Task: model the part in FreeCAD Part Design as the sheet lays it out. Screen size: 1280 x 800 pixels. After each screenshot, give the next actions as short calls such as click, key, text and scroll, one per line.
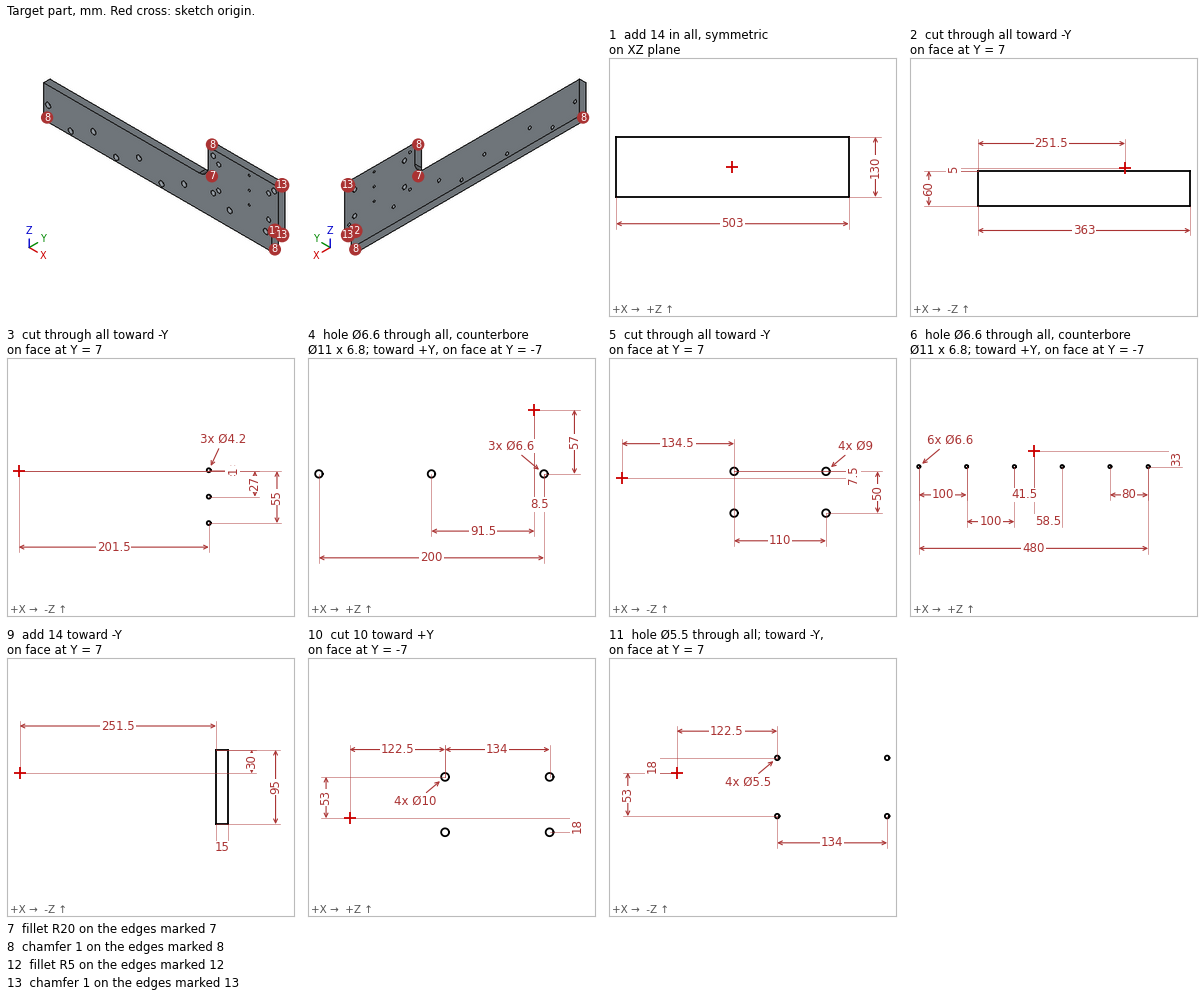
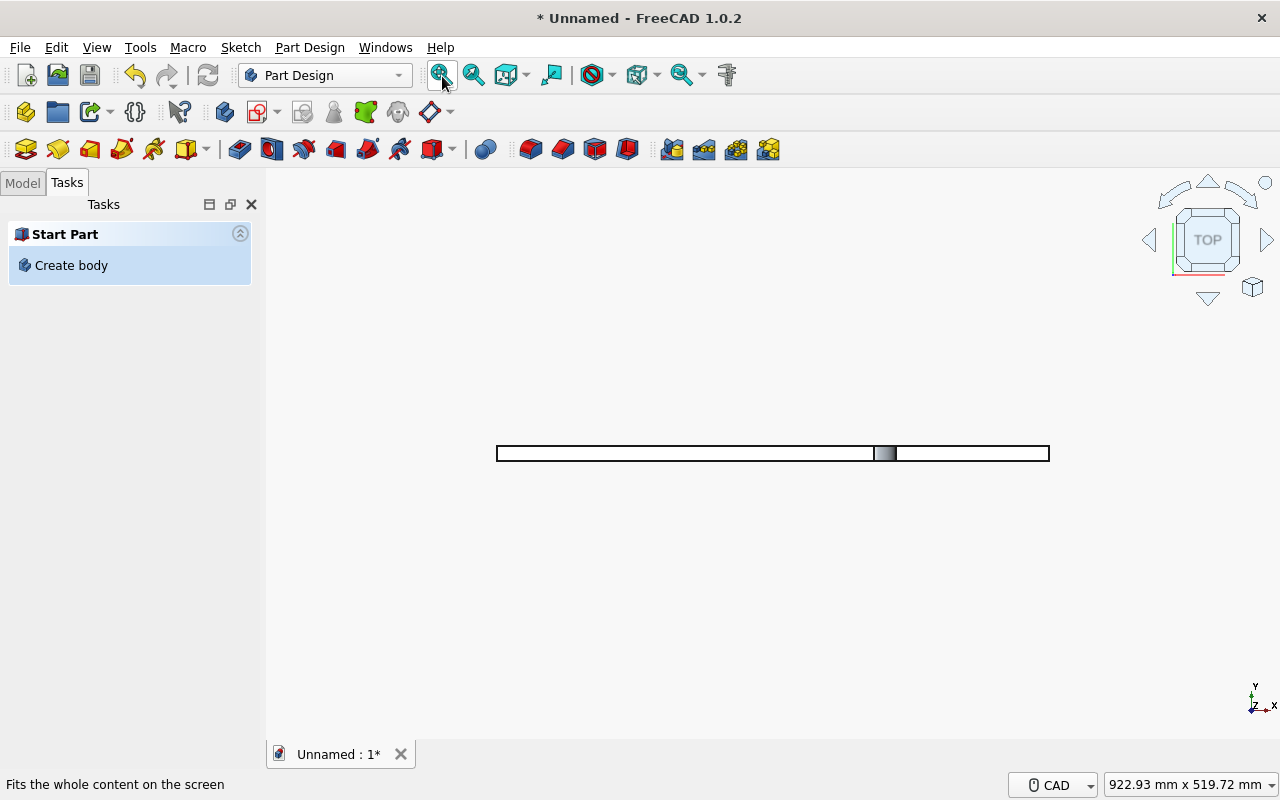
click(896, 452)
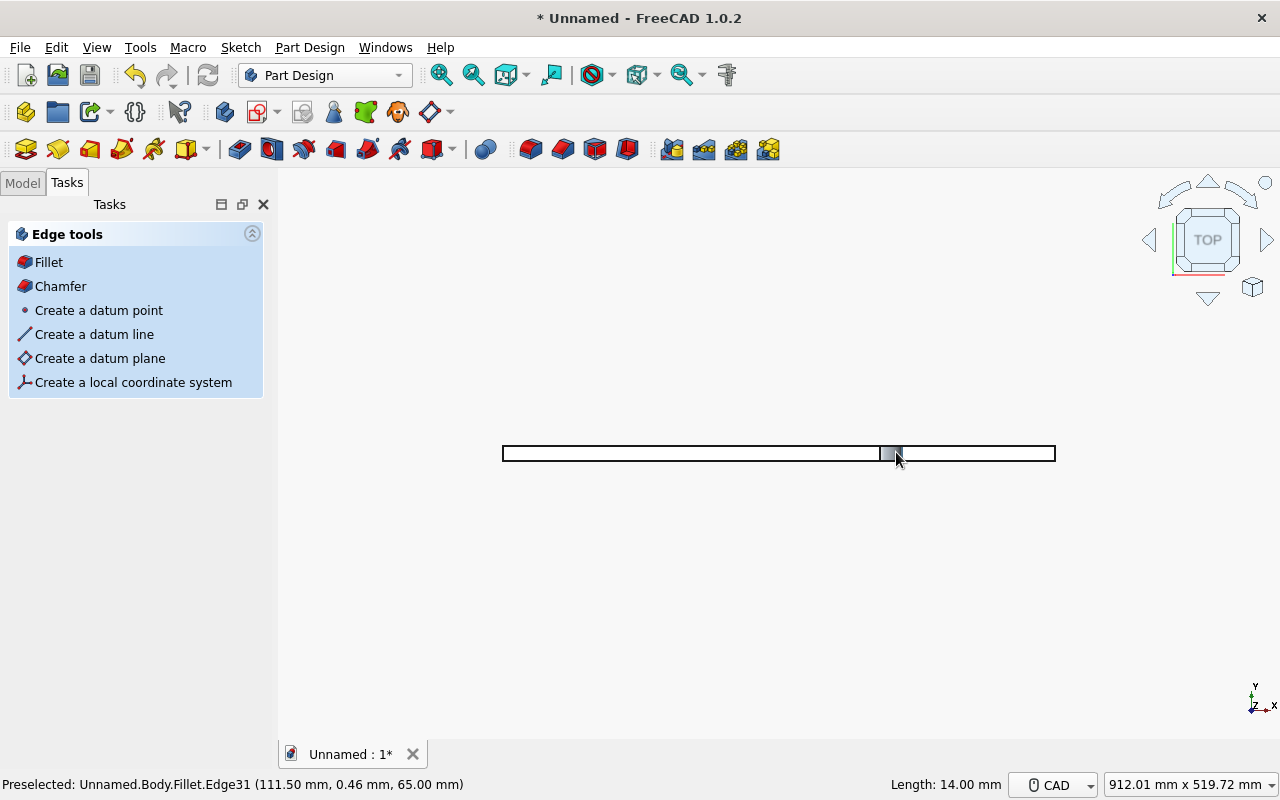
scroll(503, 452, up, 5)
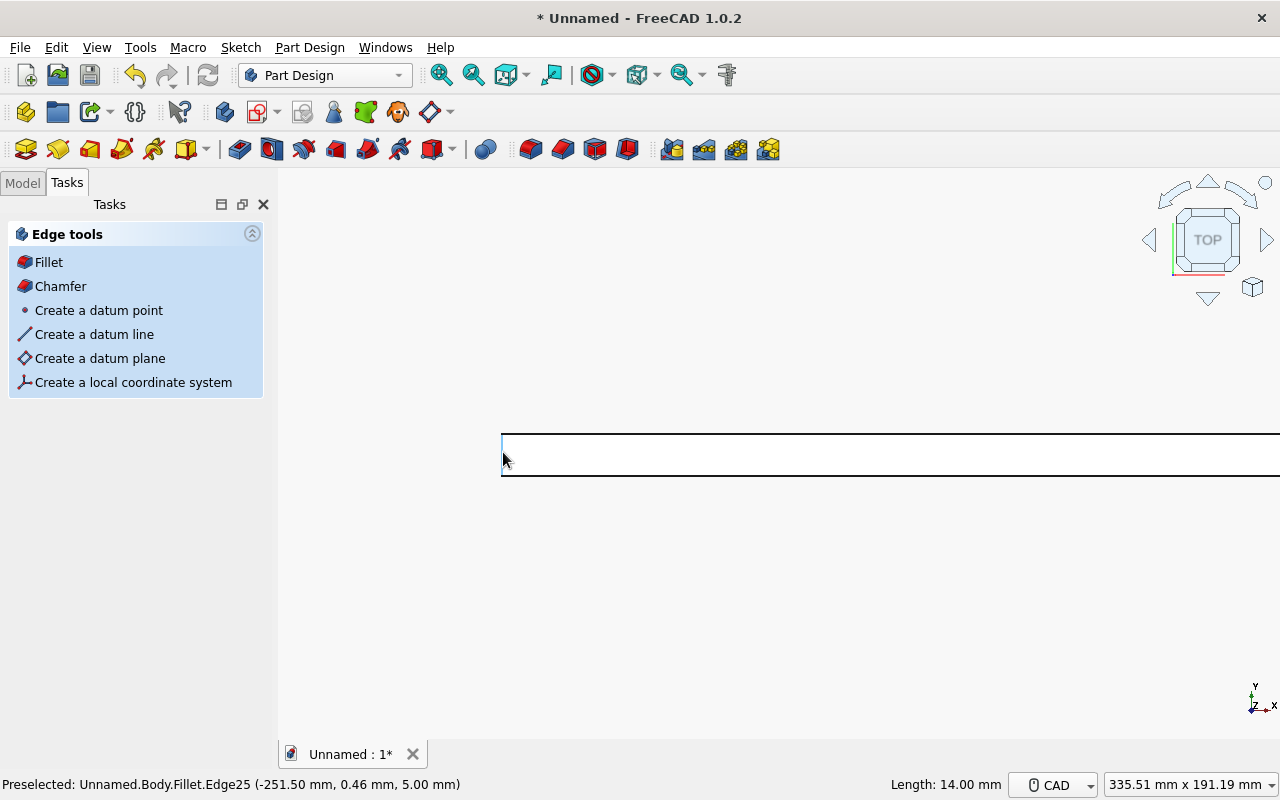
key(v)
key(f)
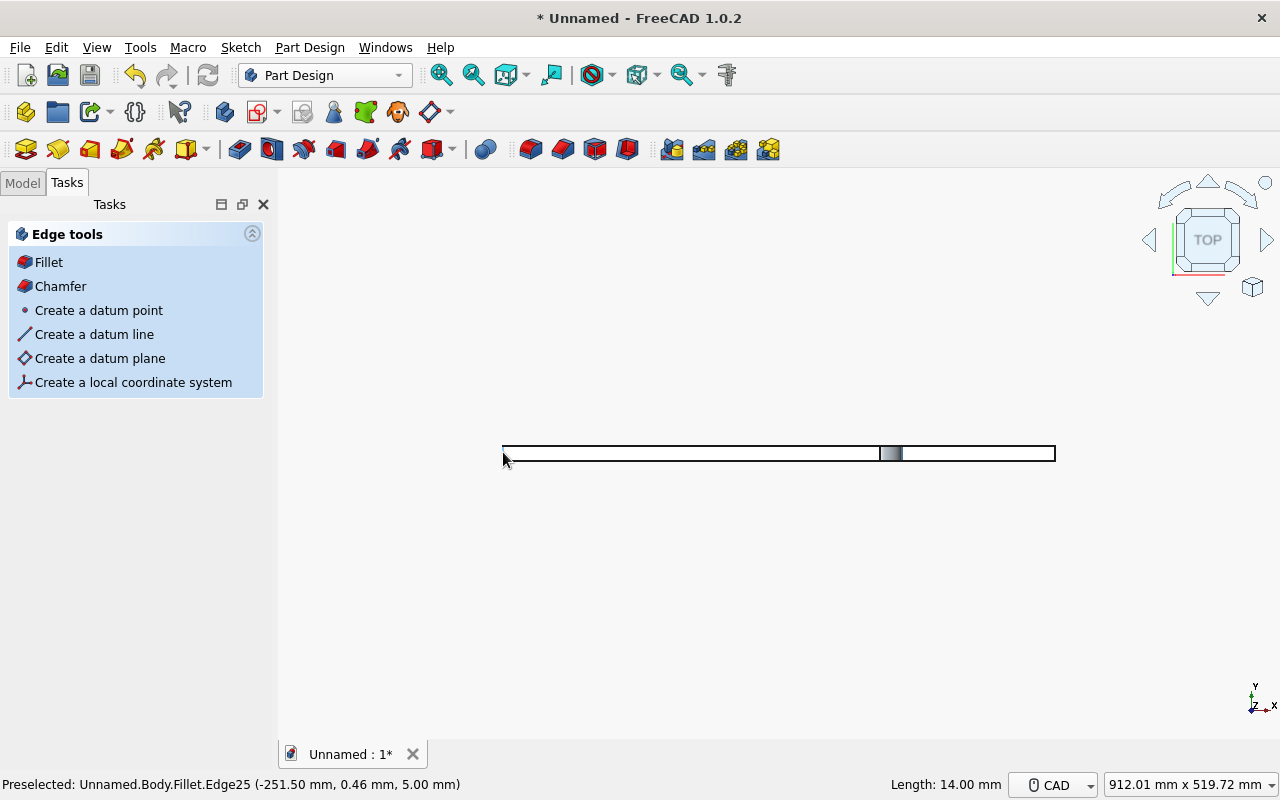
key(0)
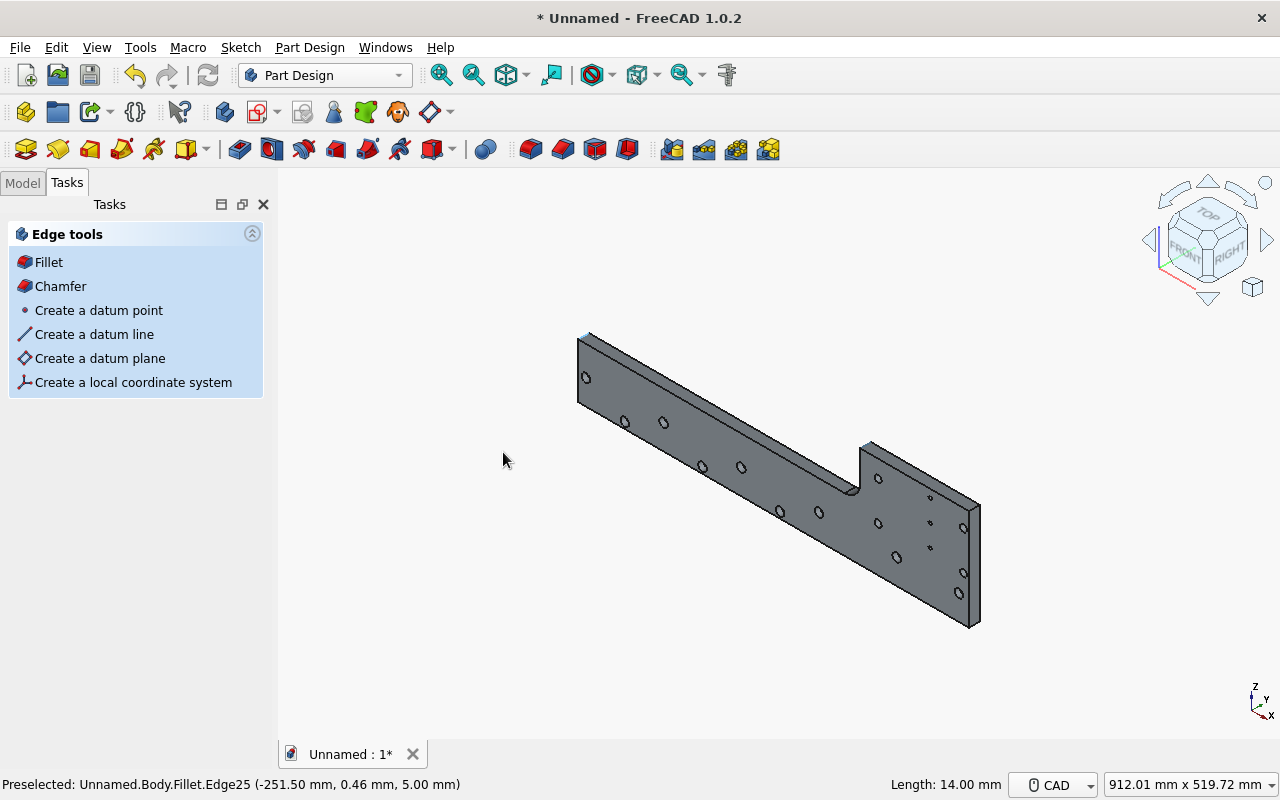
scroll(584, 398, up, 5)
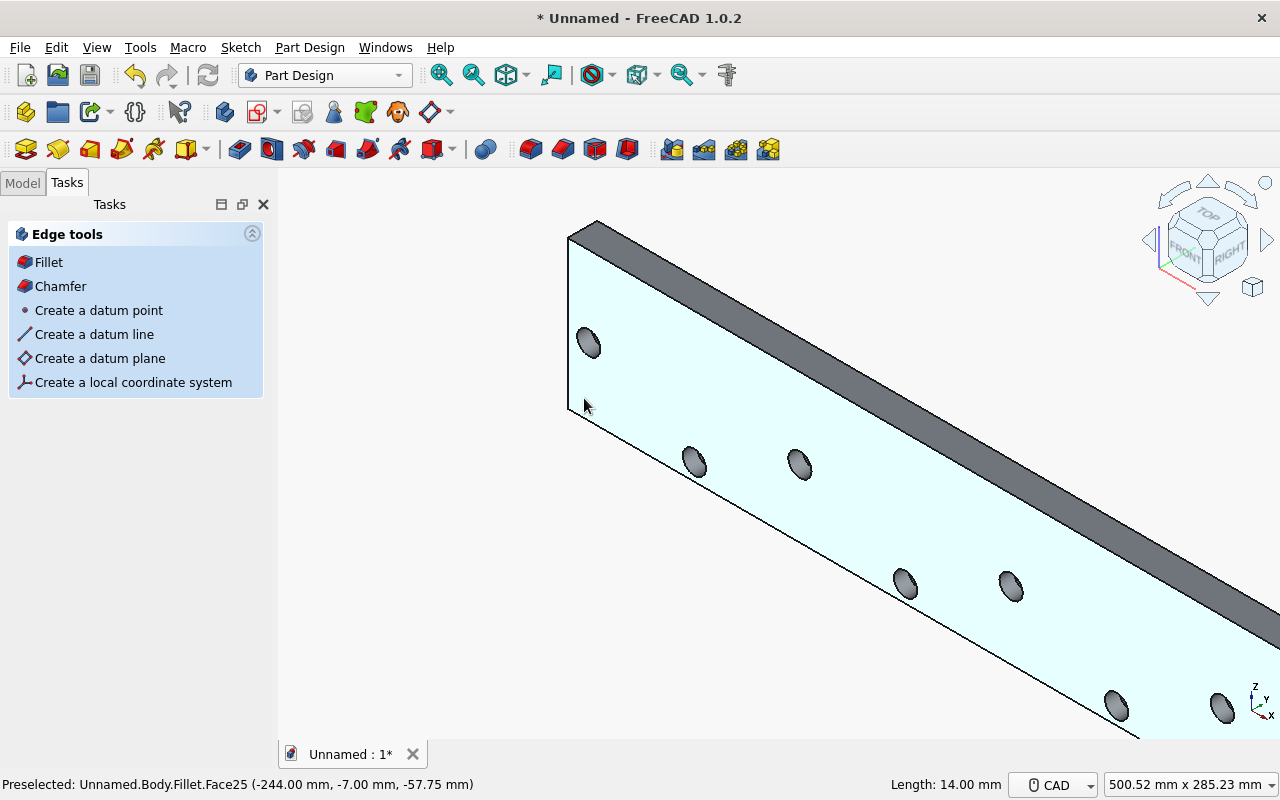
key(v)
key(f)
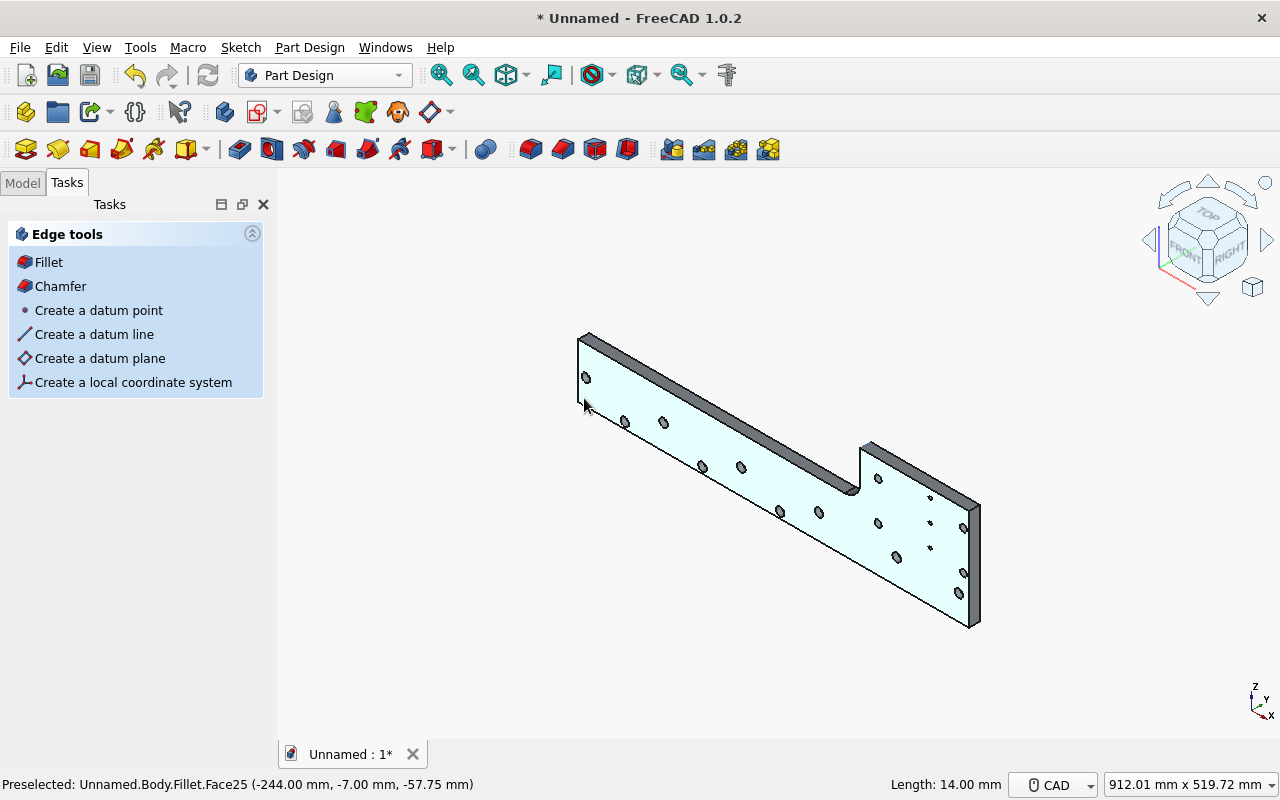
key(1)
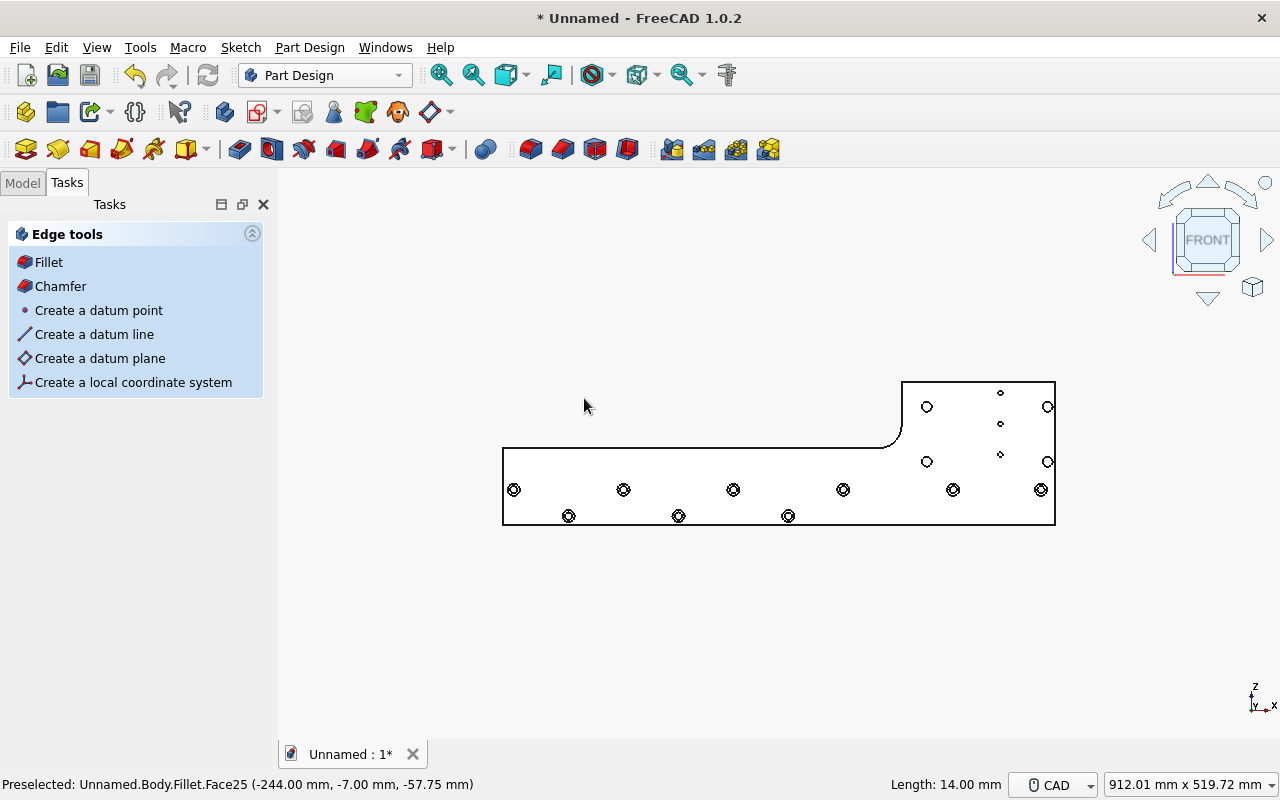
scroll(503, 524, up, 5)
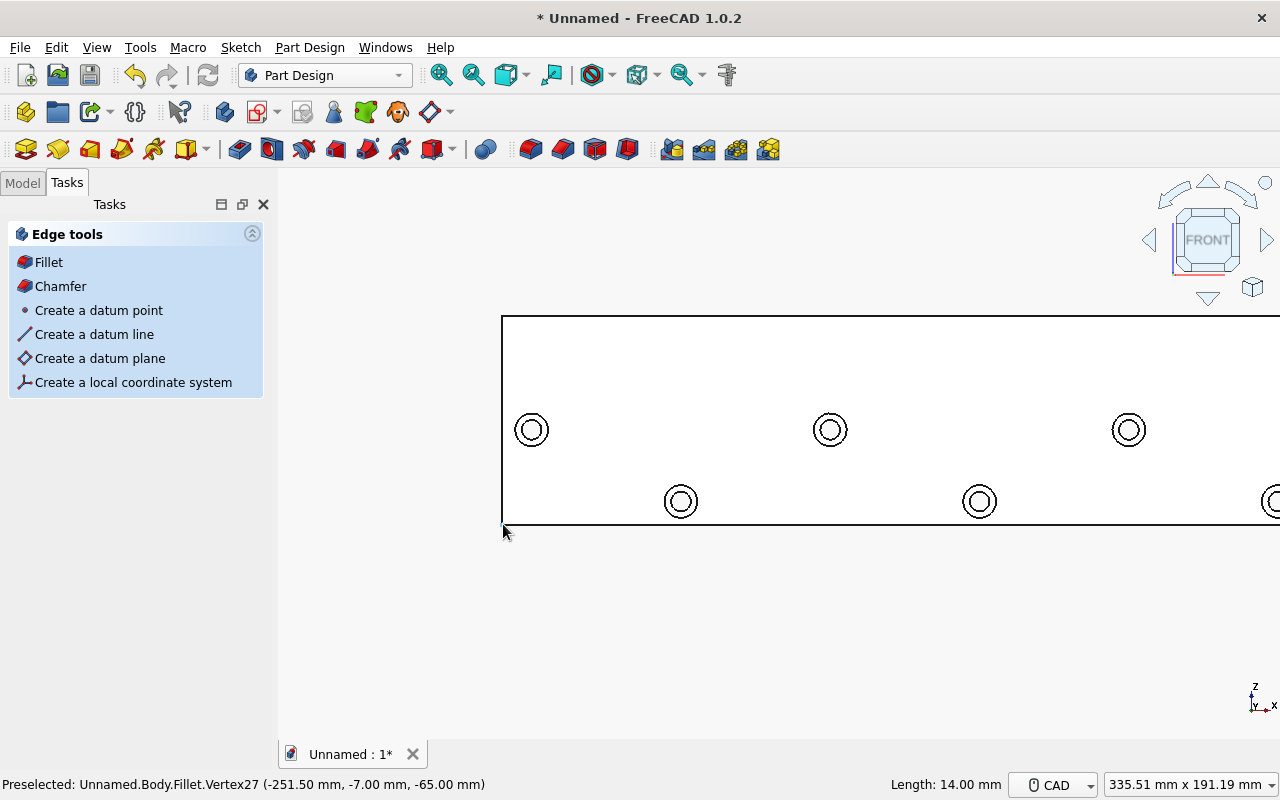
key(v)
key(f)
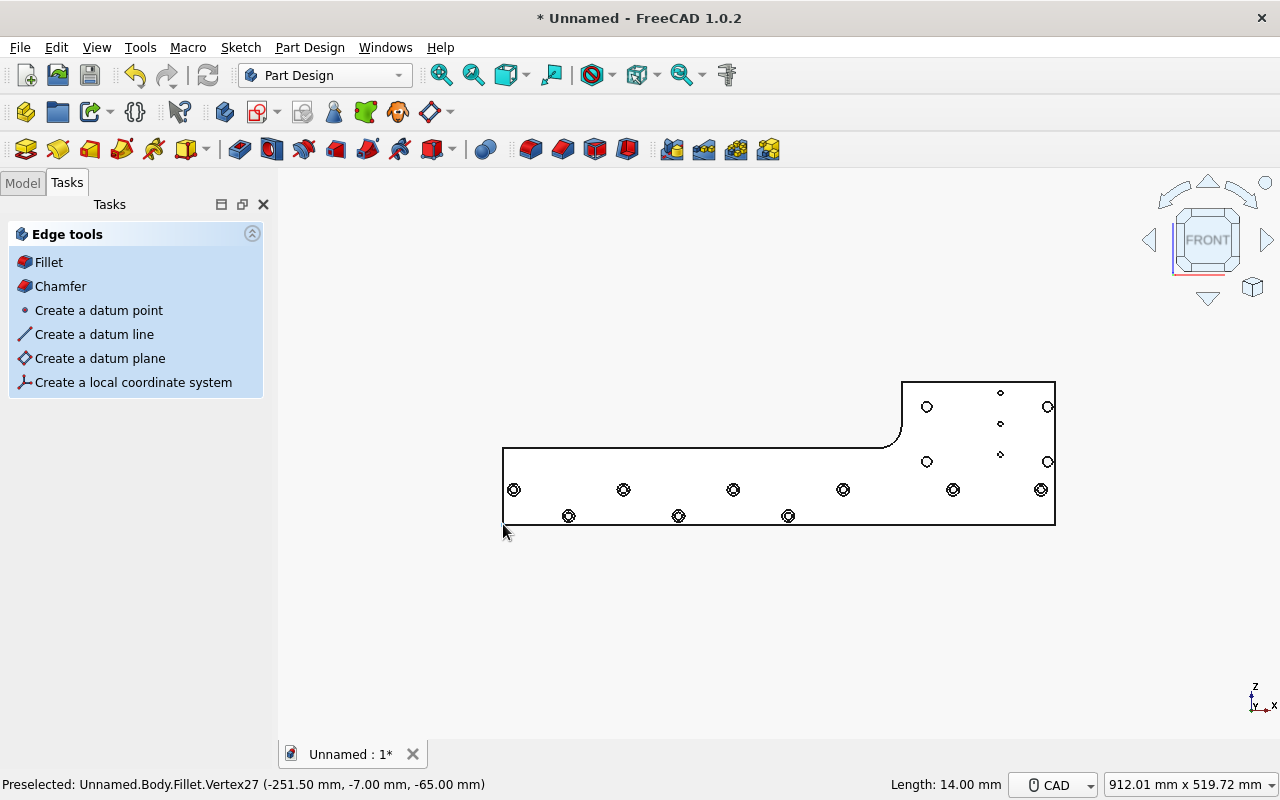
key(3)